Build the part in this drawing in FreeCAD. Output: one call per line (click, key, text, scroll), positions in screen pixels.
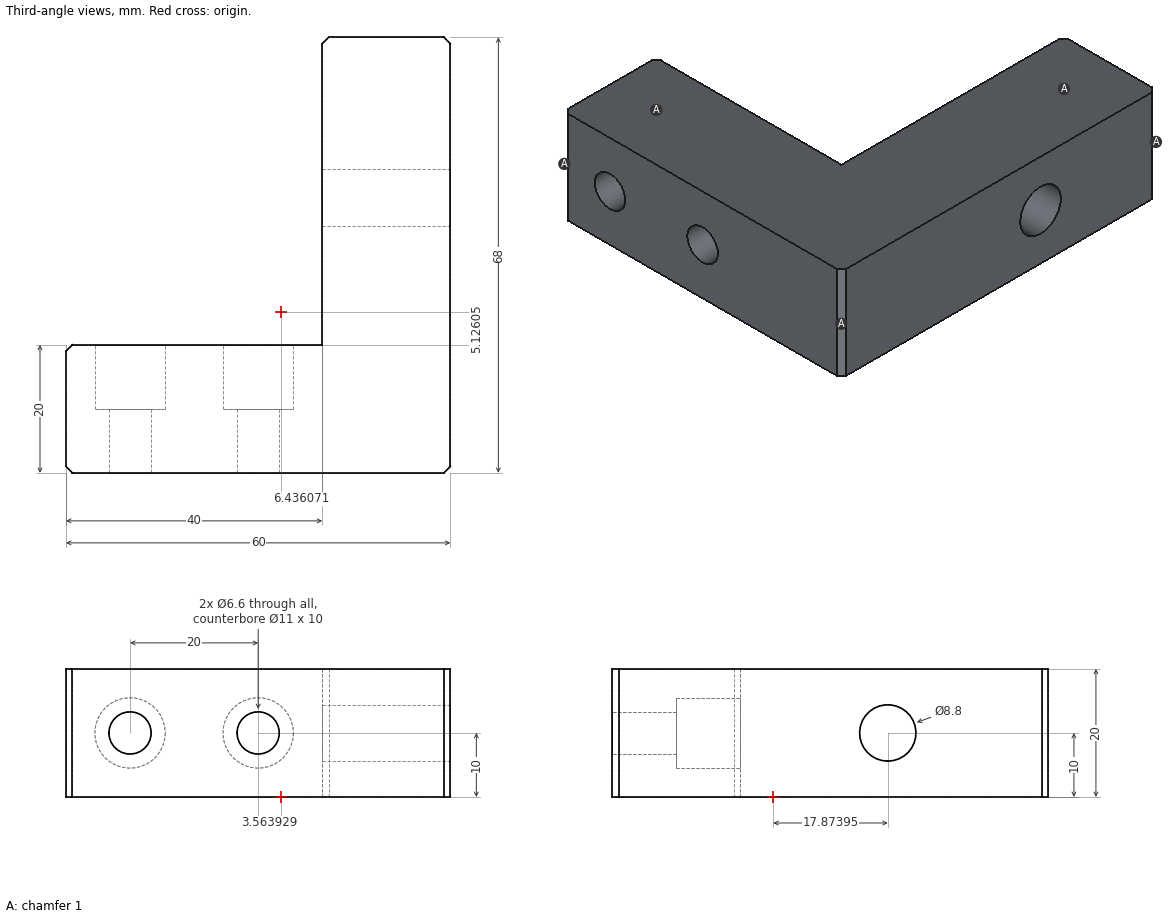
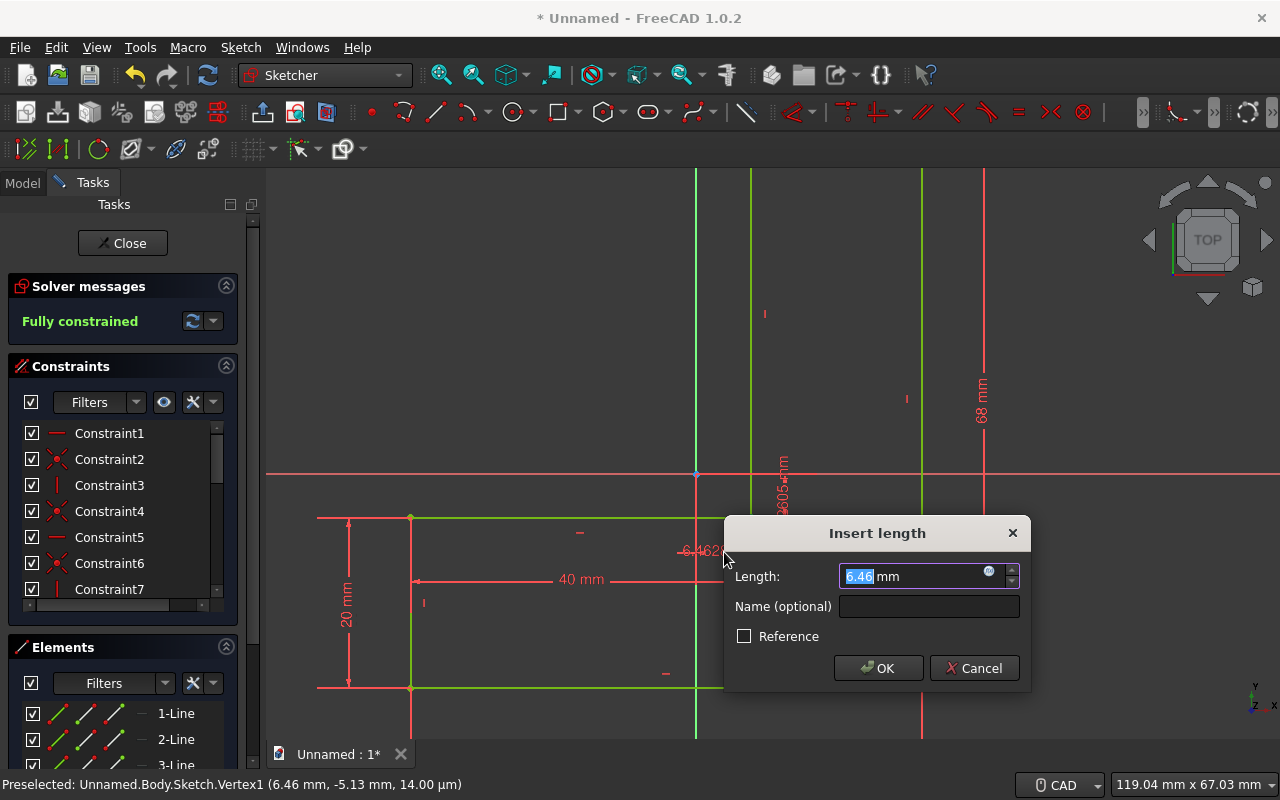
text(6.436071)
key(Return)
key(Escape)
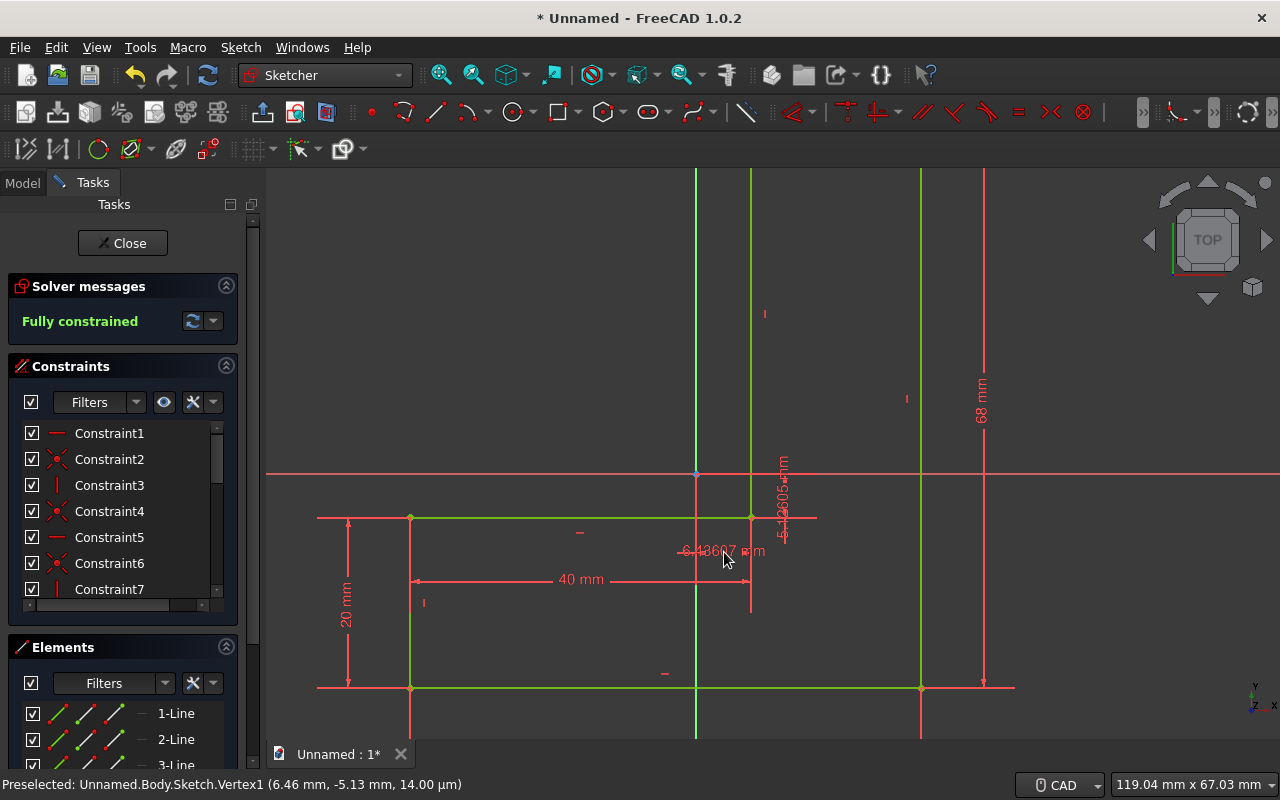
click(123, 243)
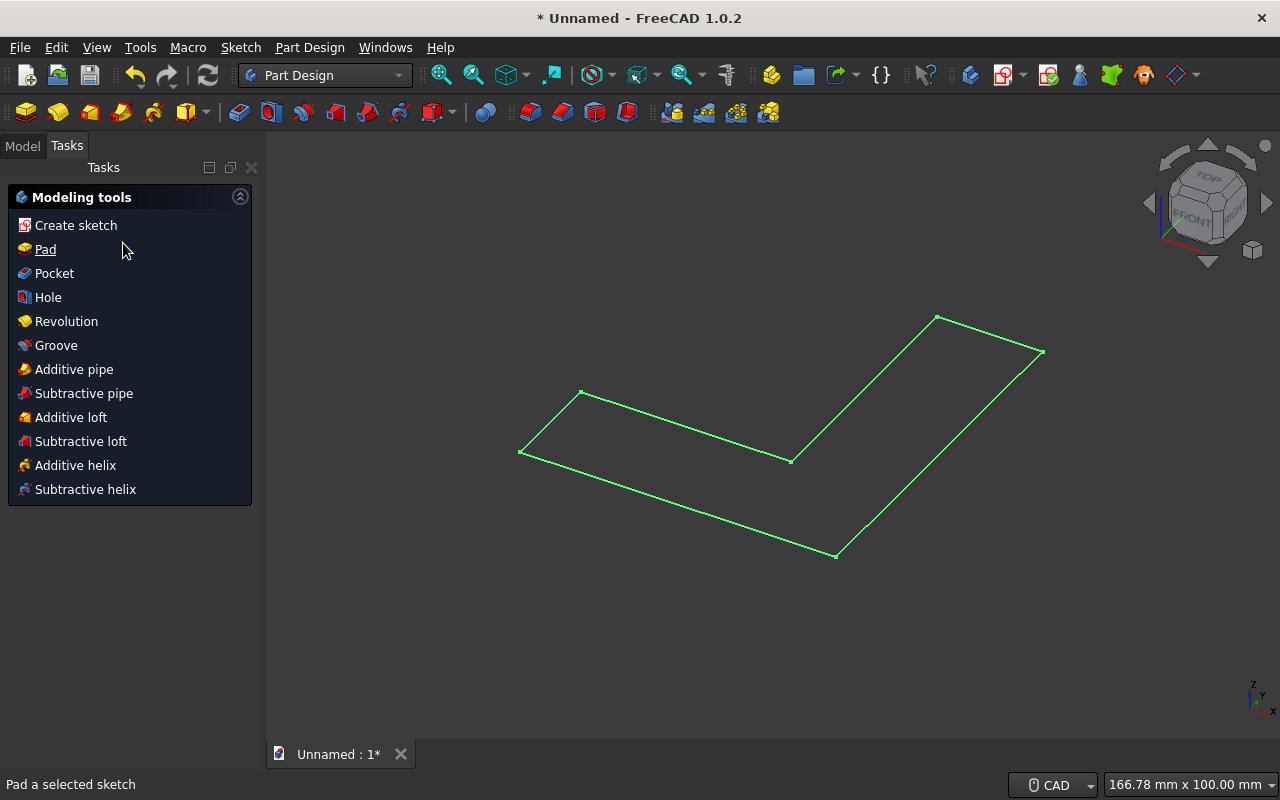
click(26, 112)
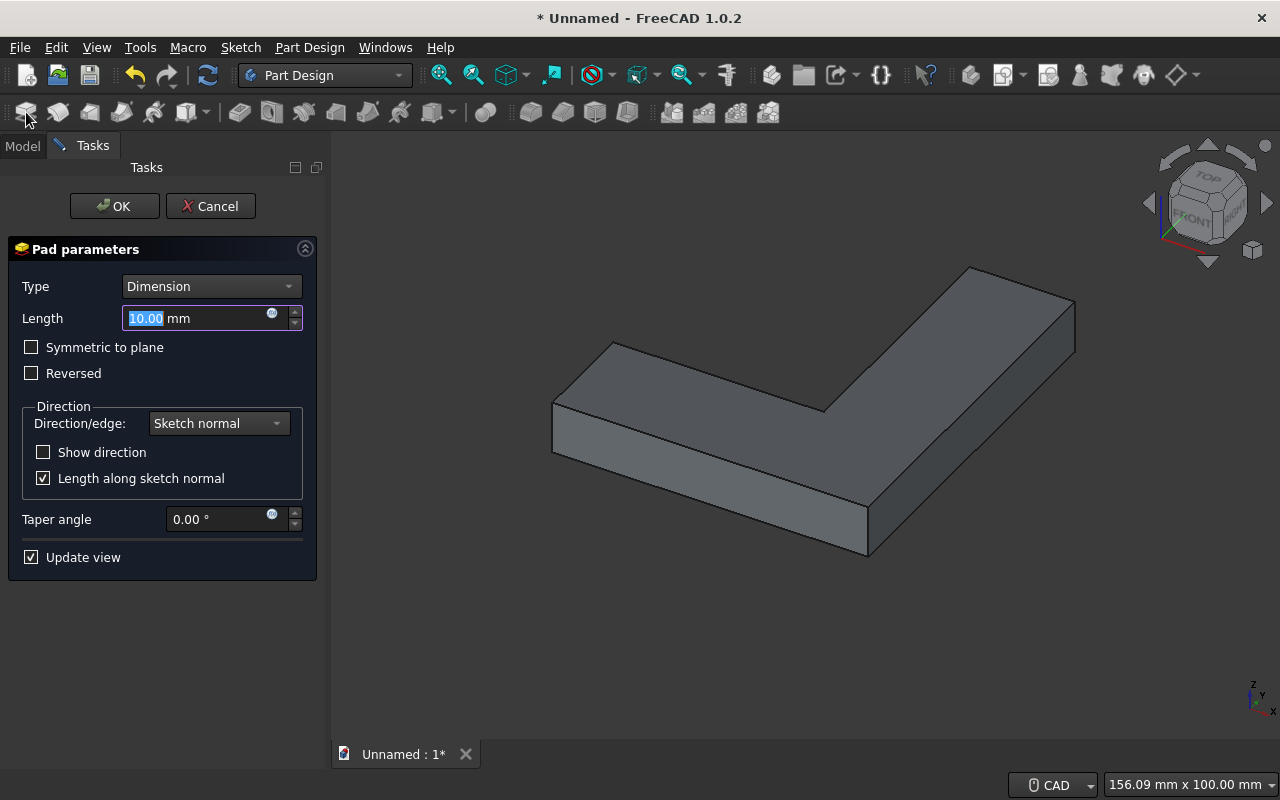
text(20)
key(Tab)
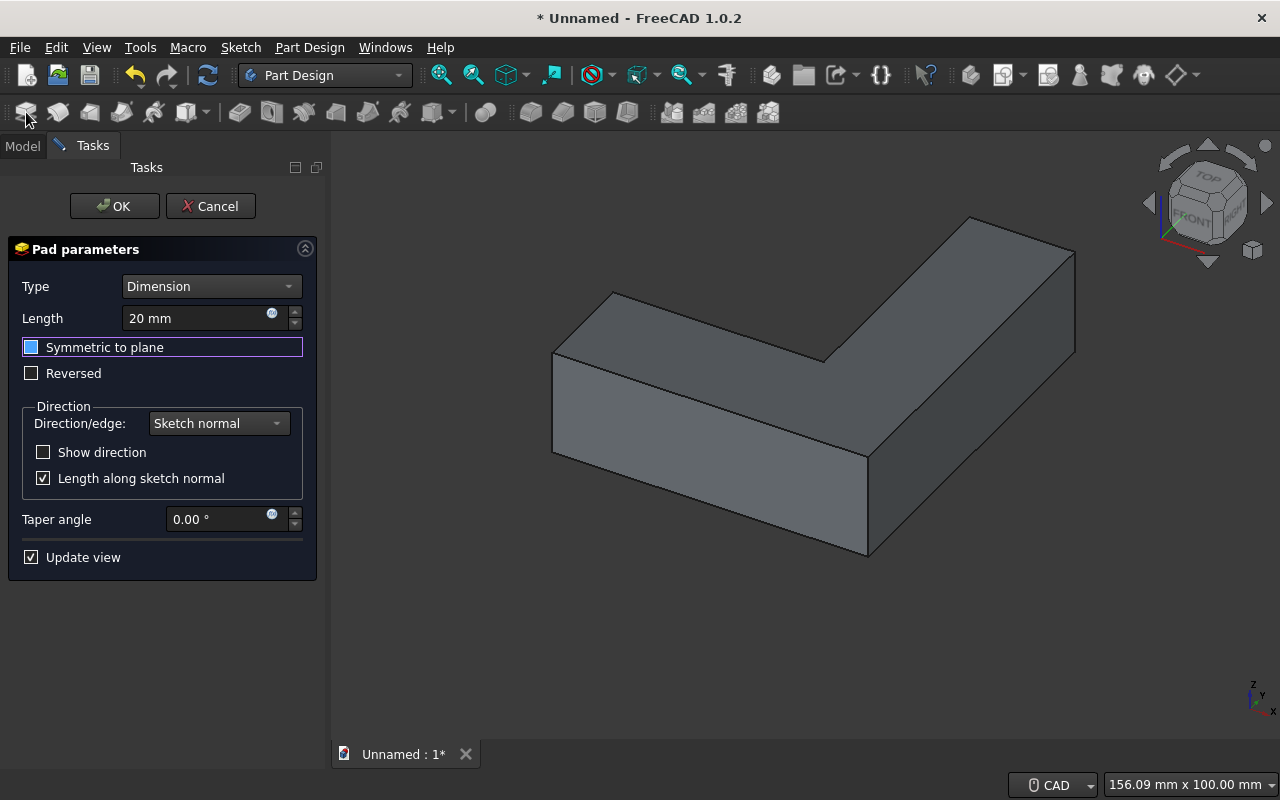
click(115, 206)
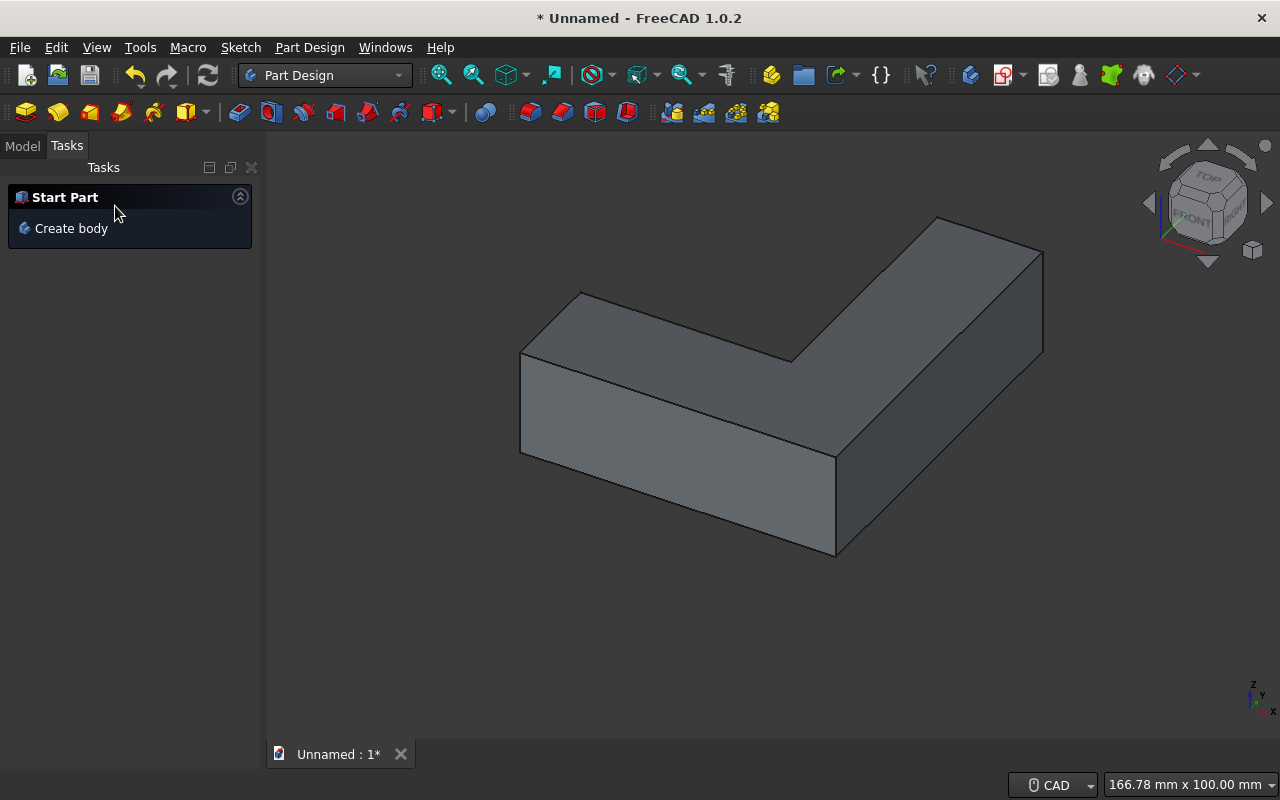
key(6)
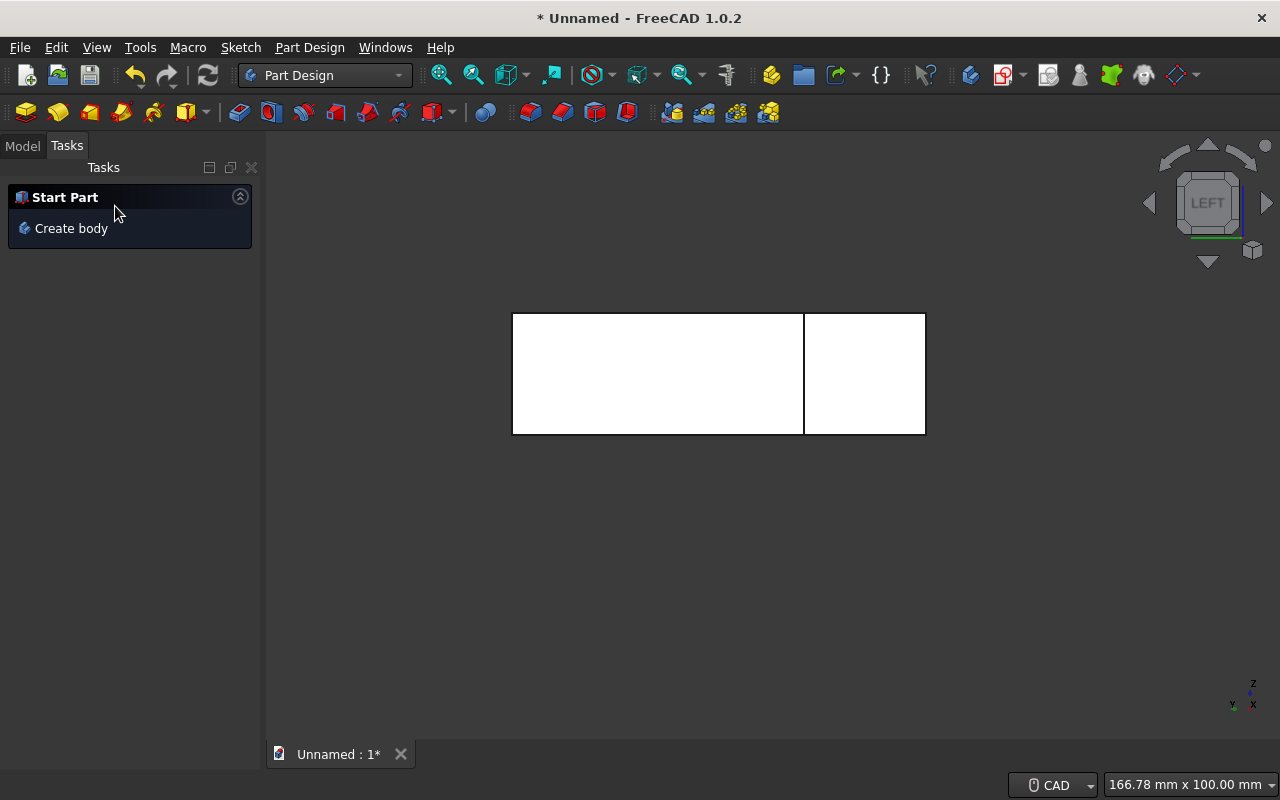
click(442, 76)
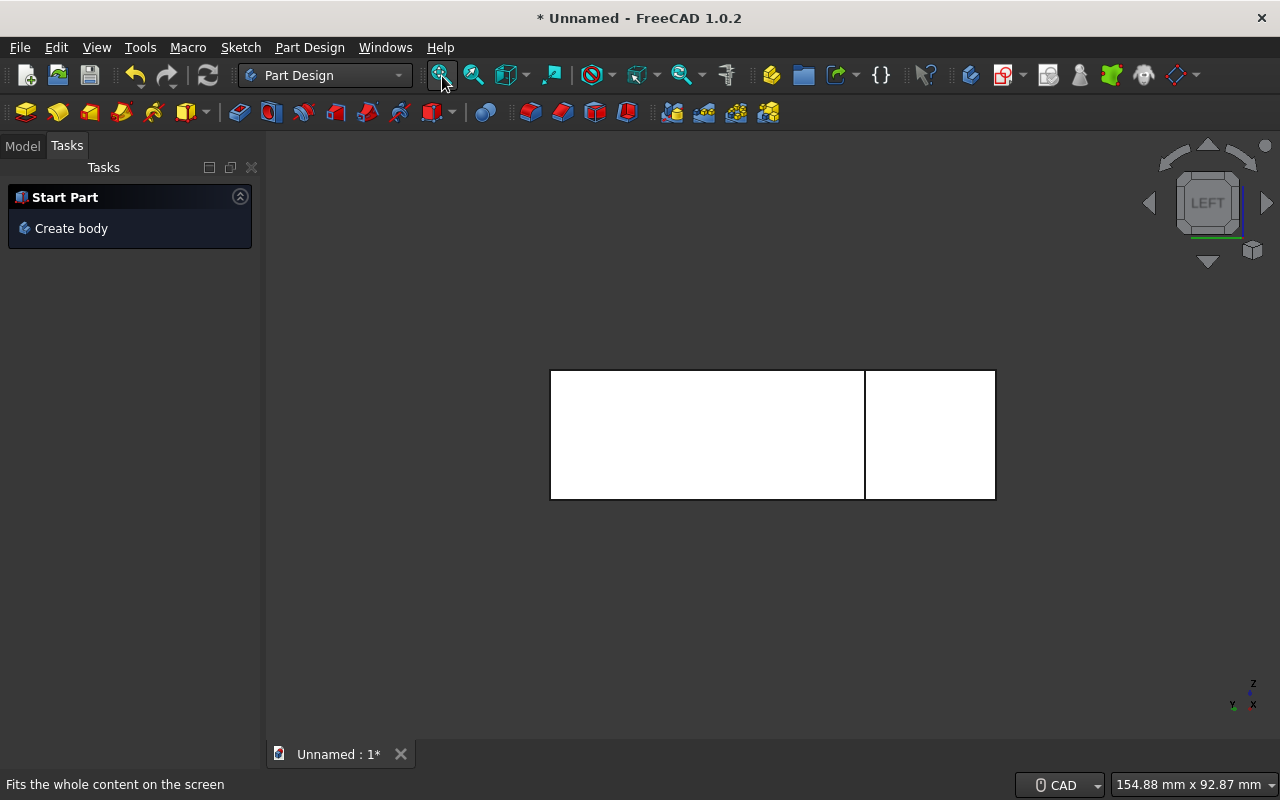
click(618, 434)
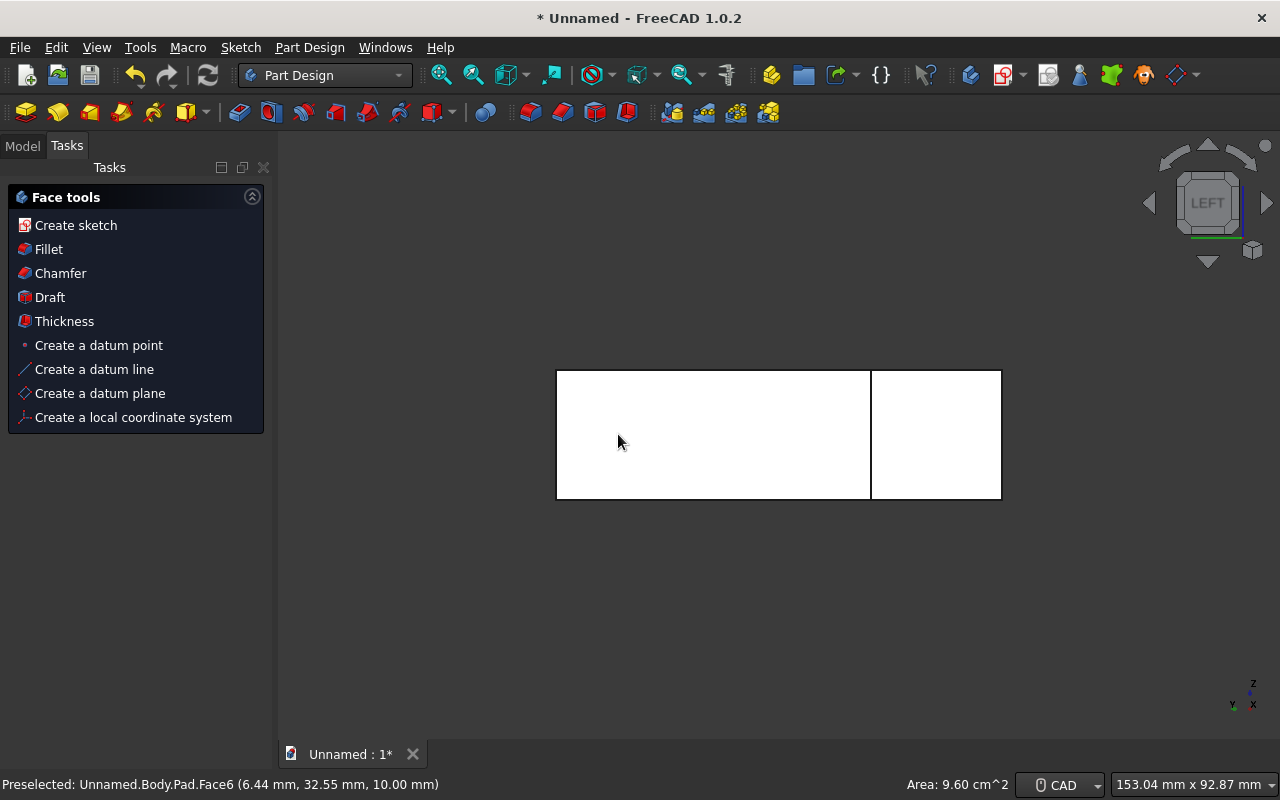
click(1004, 76)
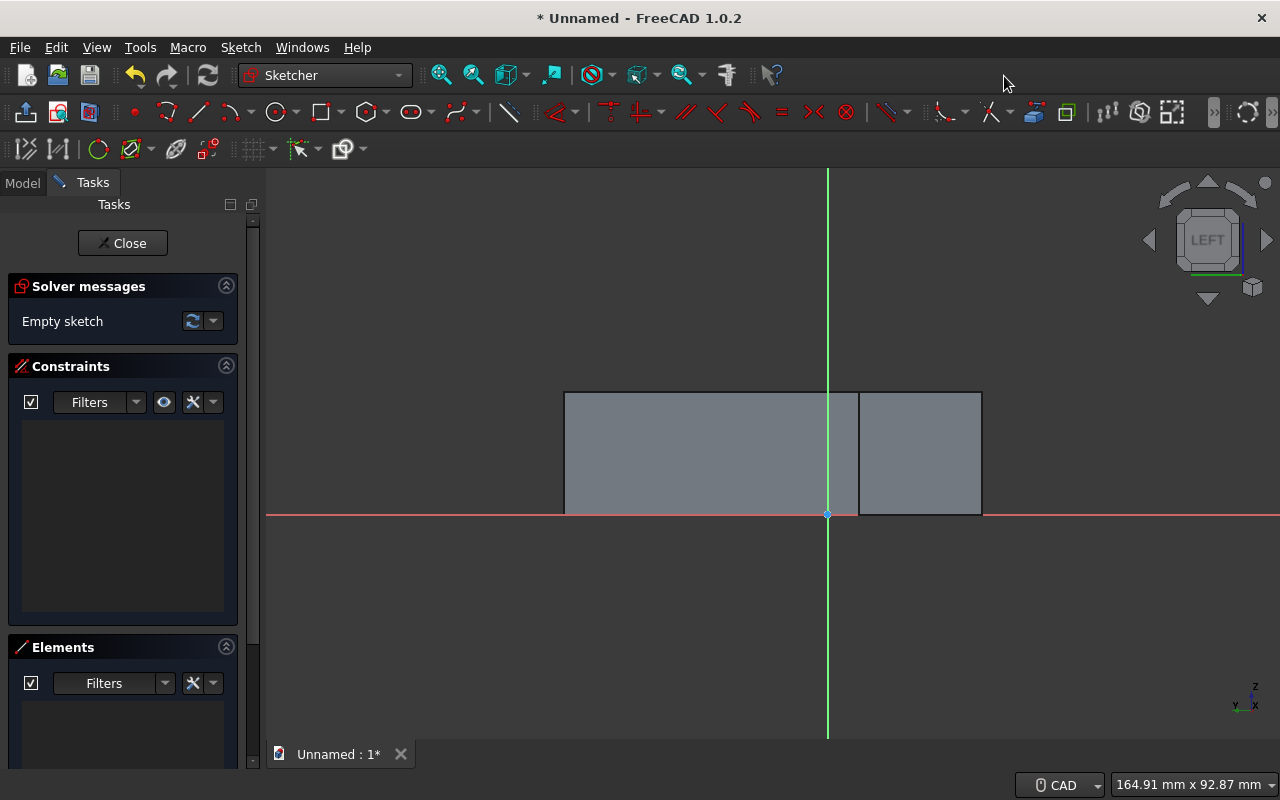
scroll(720, 454, up, 10)